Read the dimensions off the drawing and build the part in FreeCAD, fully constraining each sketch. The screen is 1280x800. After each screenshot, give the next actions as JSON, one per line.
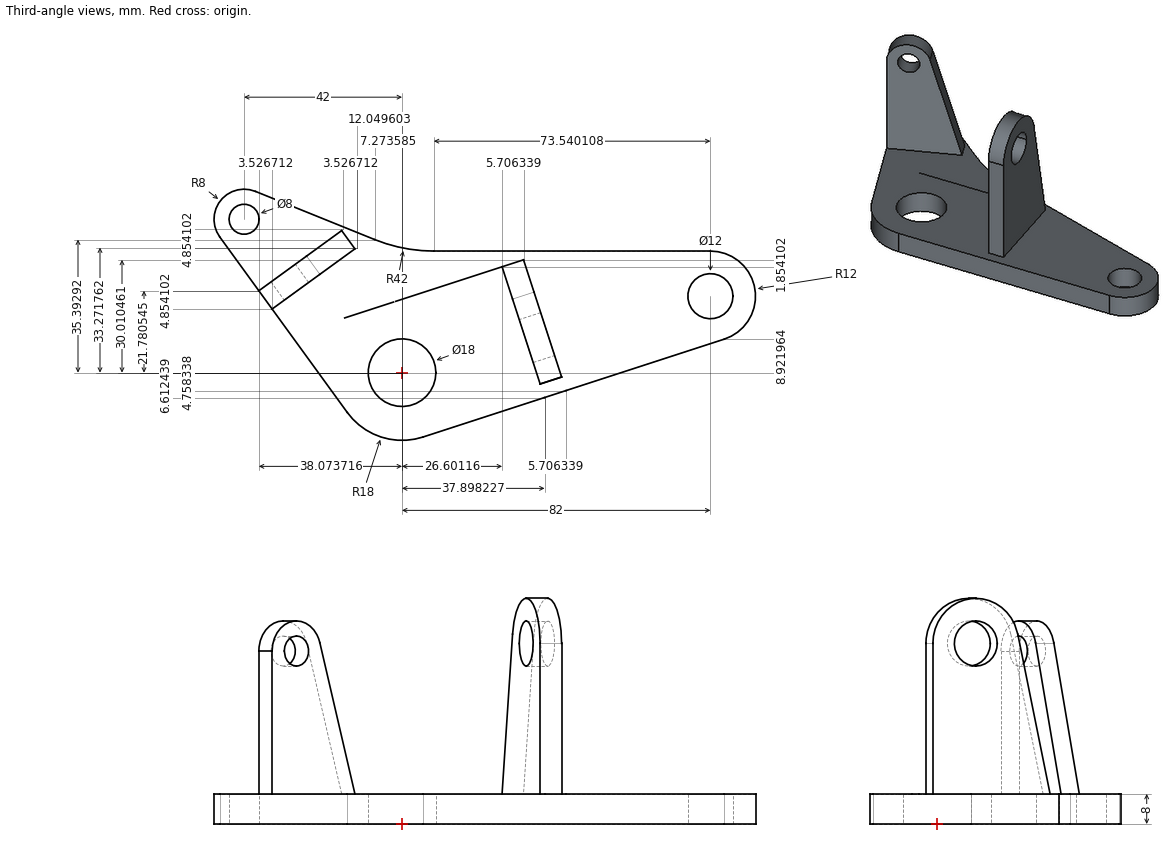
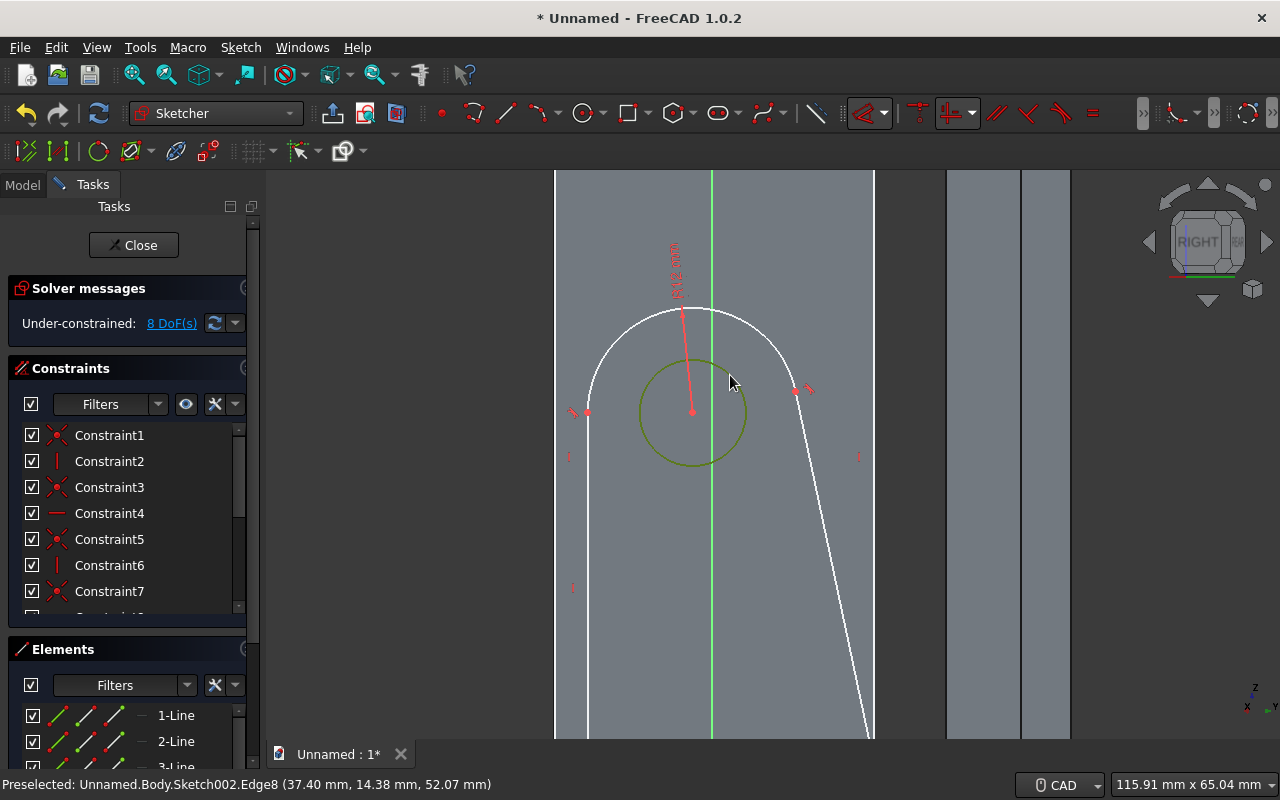
{"action": "key", "text": "k o"}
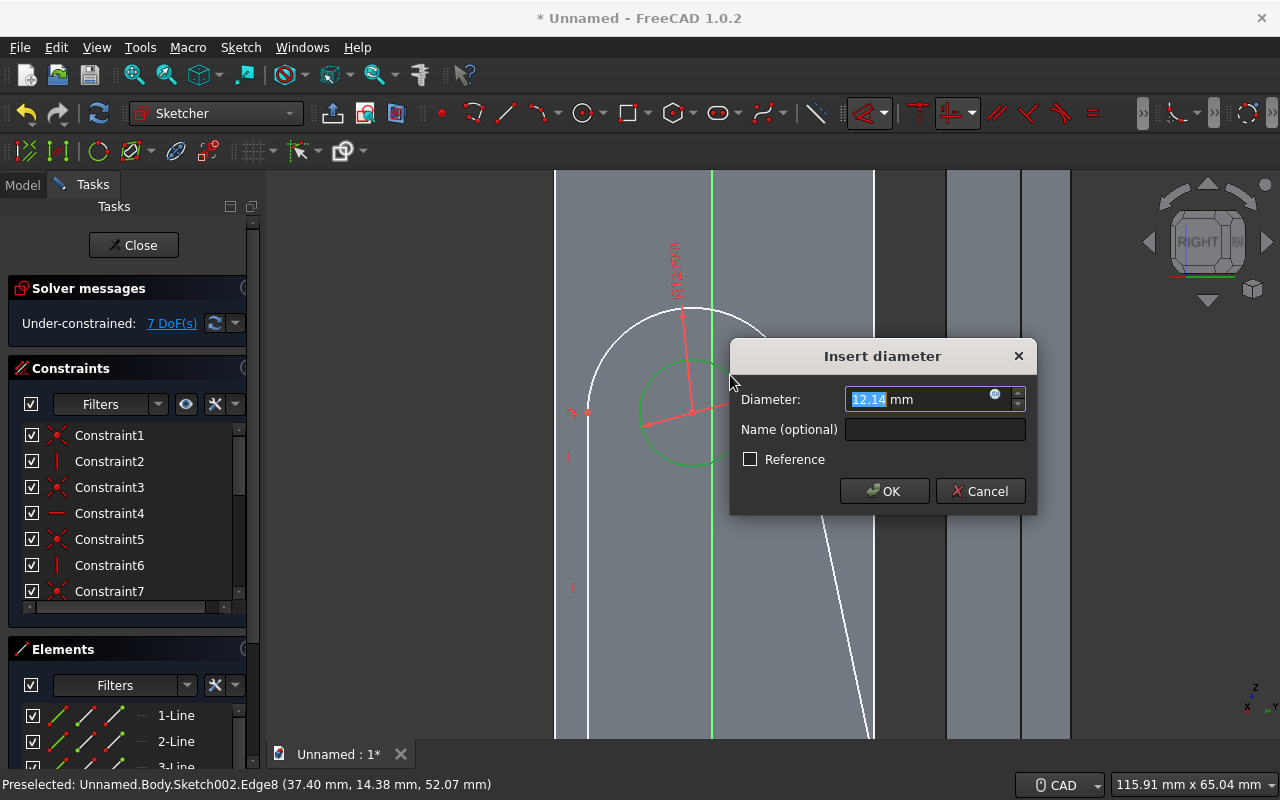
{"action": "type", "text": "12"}
{"action": "key", "text": "Return"}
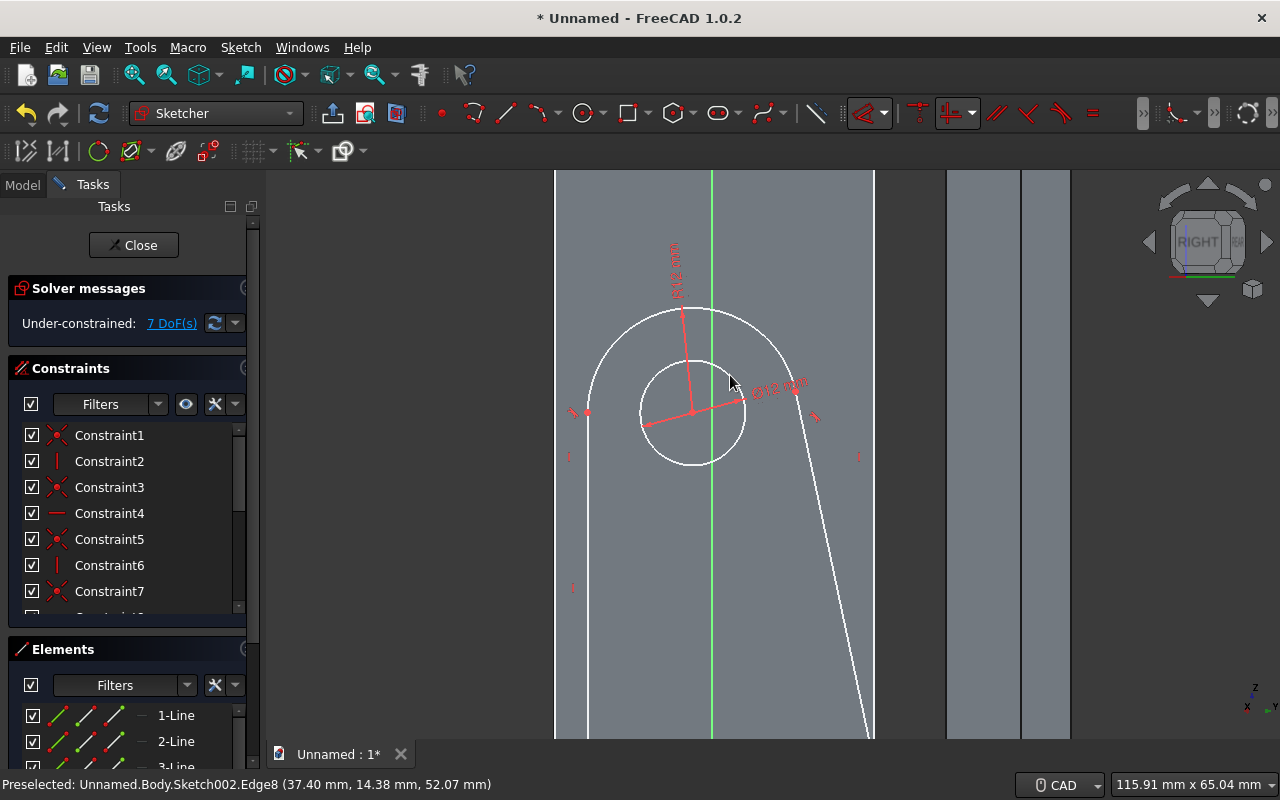
{"action": "left_click", "coordinate": [874, 579]}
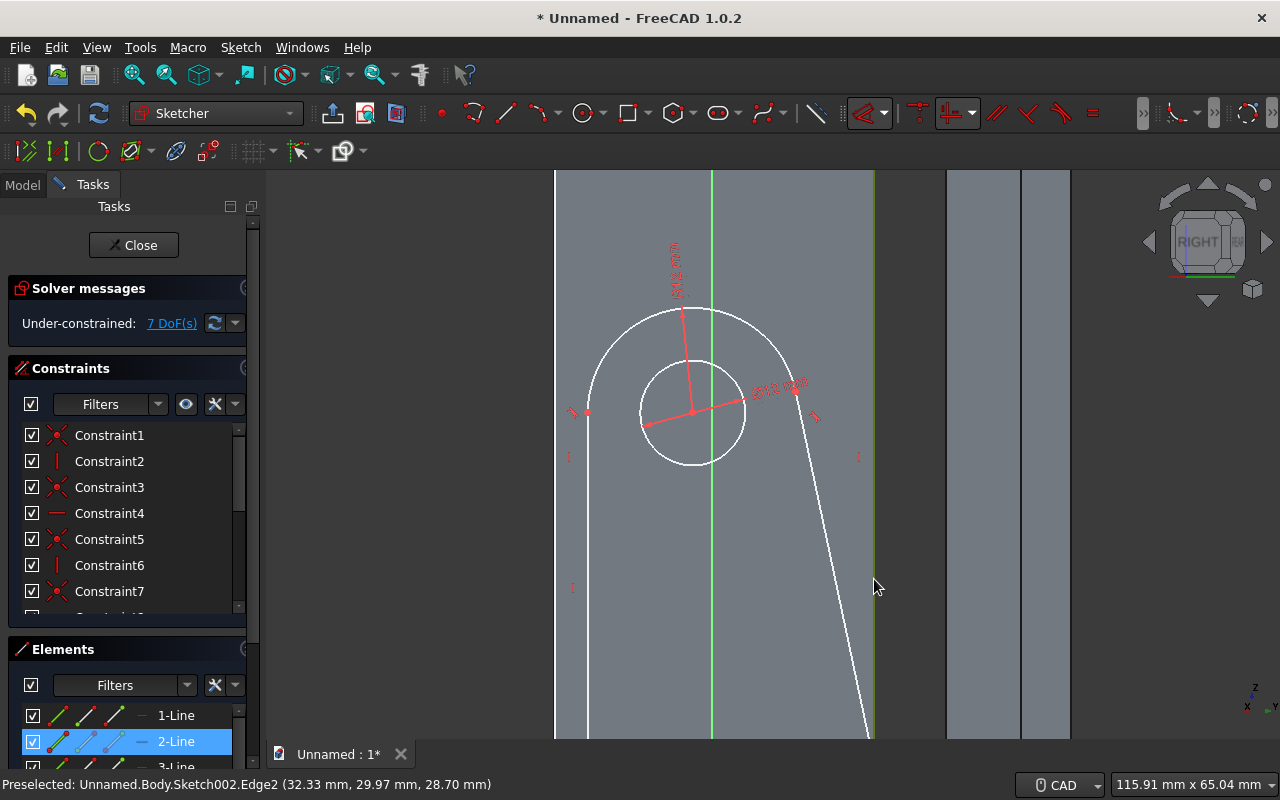
{"action": "key", "text": "i"}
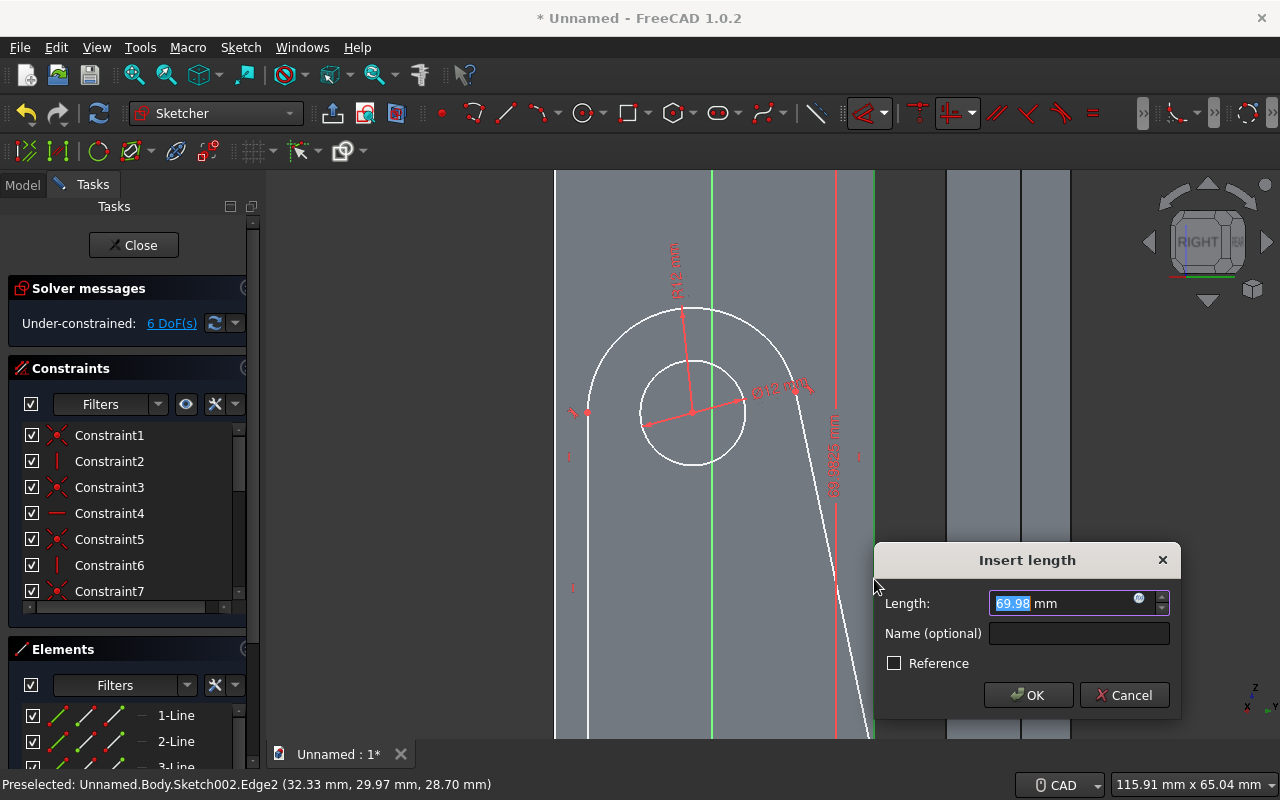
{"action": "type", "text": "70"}
{"action": "key", "text": "Return"}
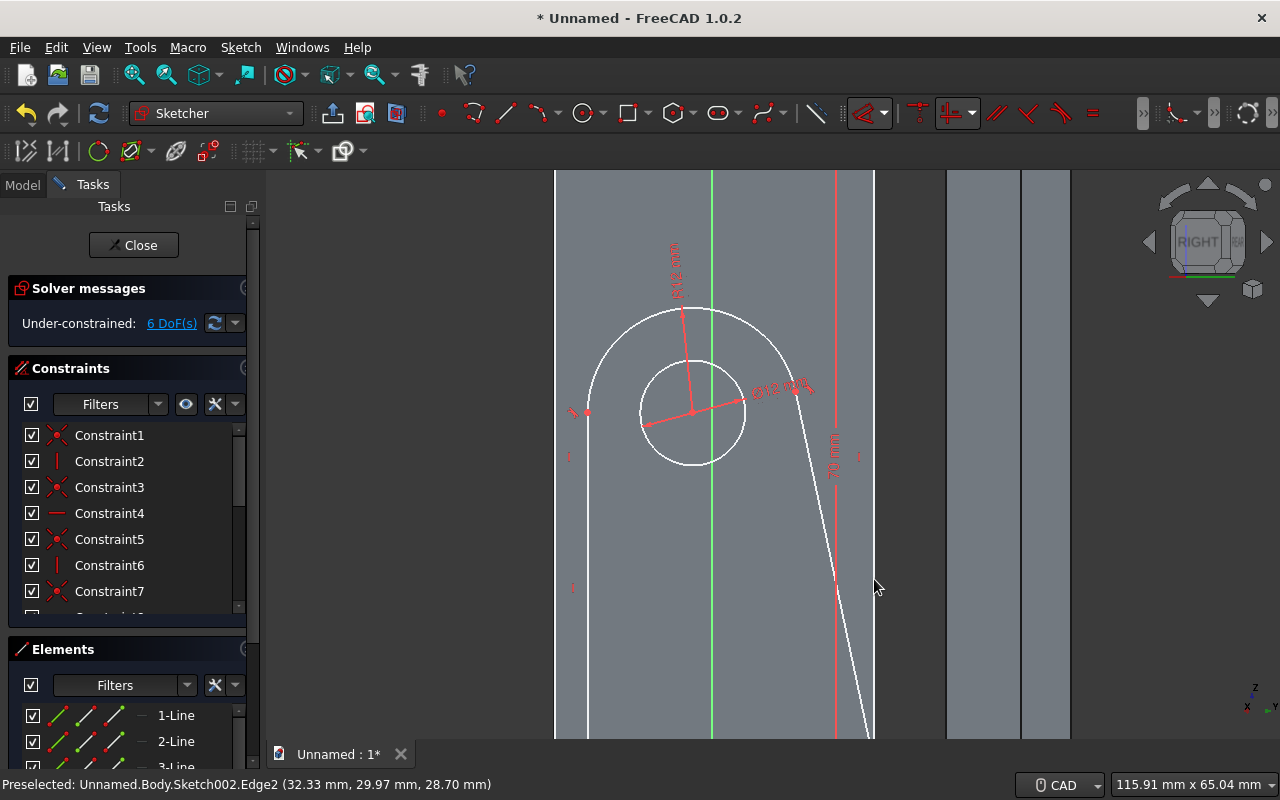
{"action": "left_click", "coordinate": [555, 334]}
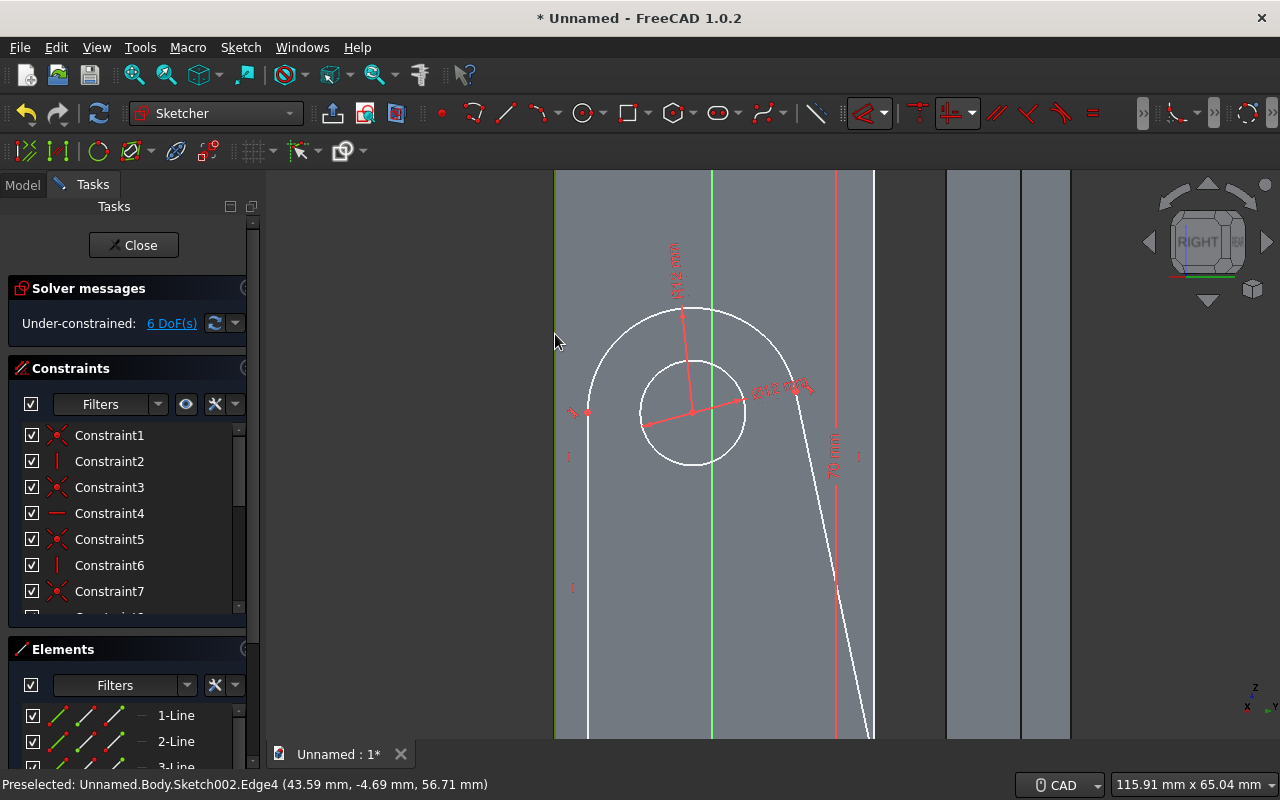
{"action": "key", "text": "i"}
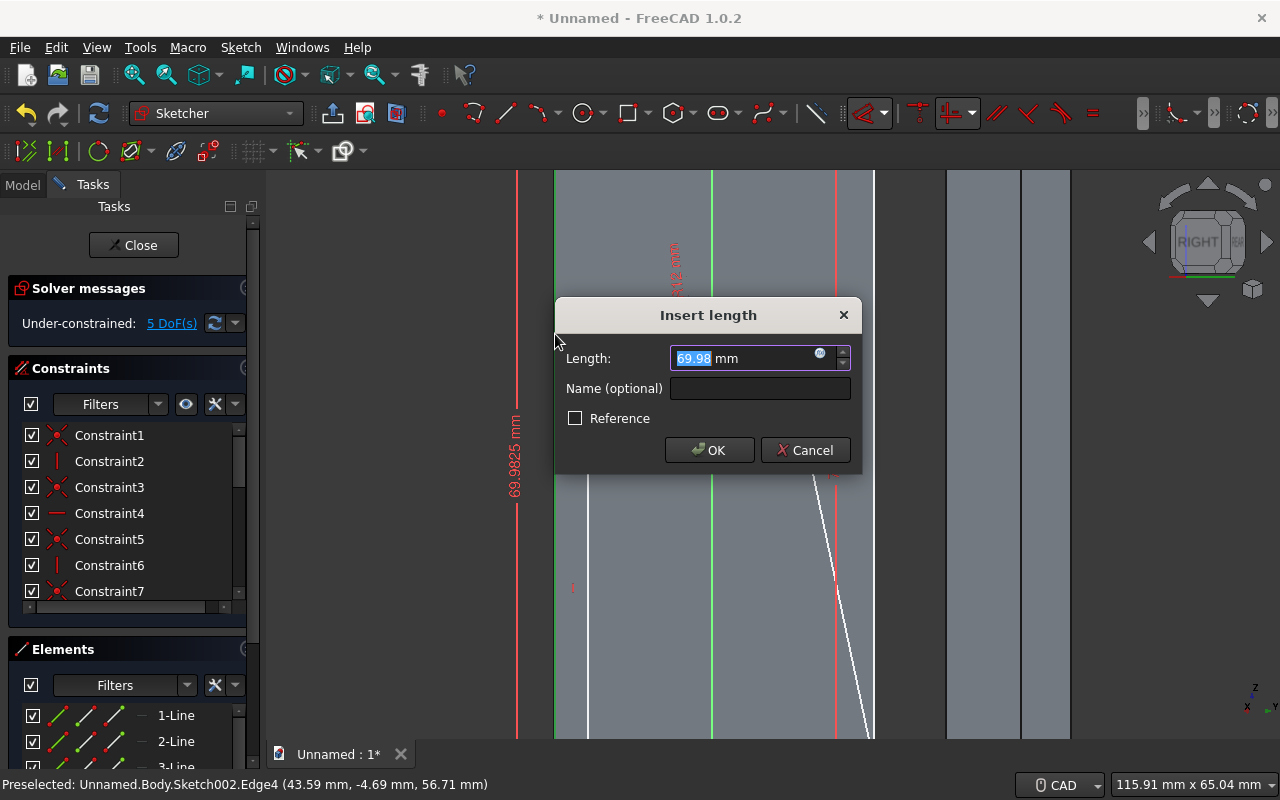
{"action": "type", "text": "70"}
{"action": "key", "text": "Return"}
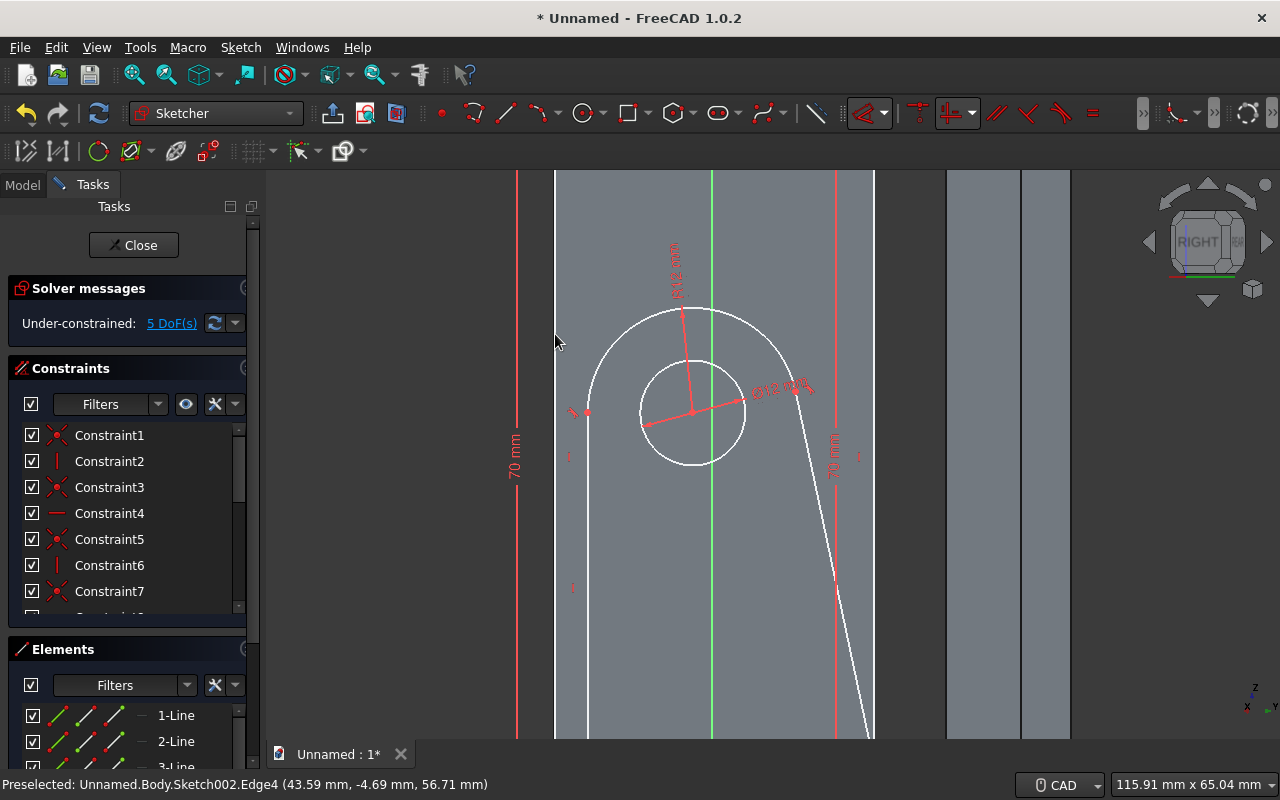
{"action": "left_click", "coordinate": [588, 658]}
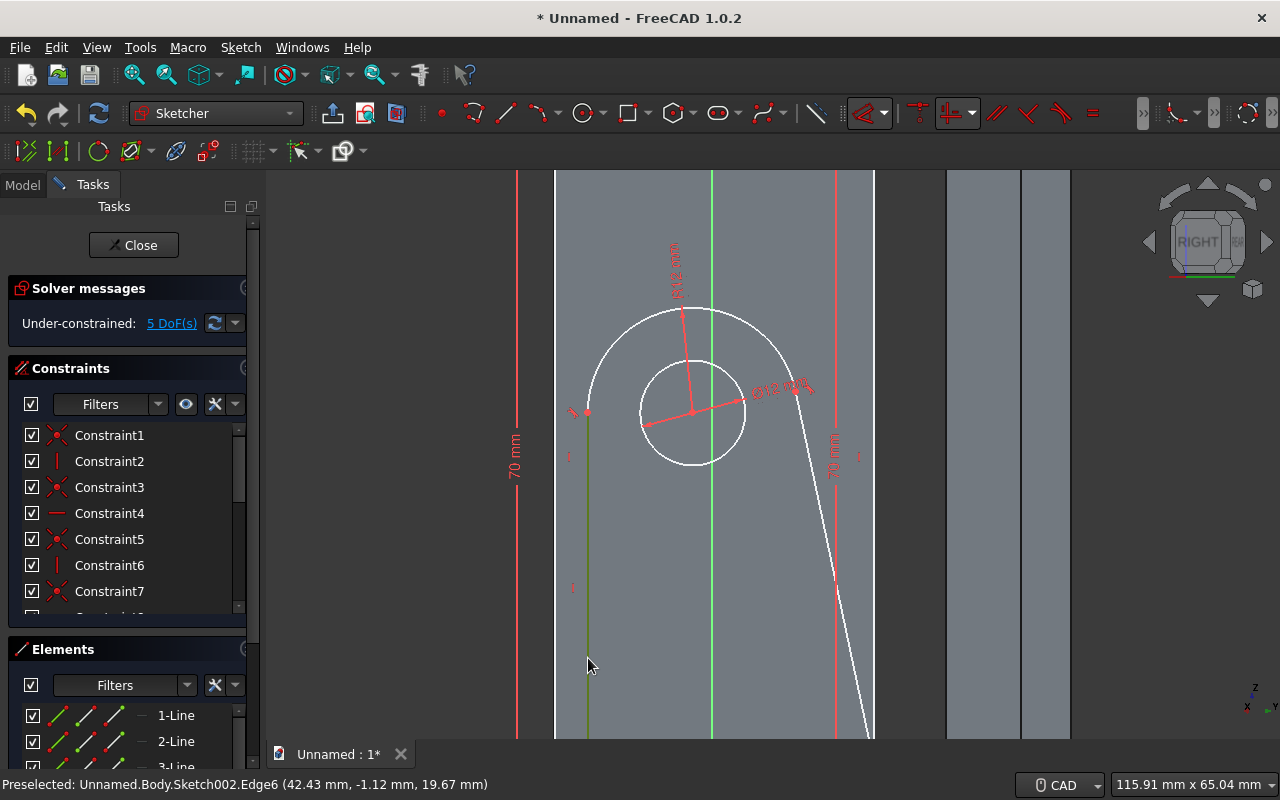
{"action": "left_click", "coordinate": [886, 114]}